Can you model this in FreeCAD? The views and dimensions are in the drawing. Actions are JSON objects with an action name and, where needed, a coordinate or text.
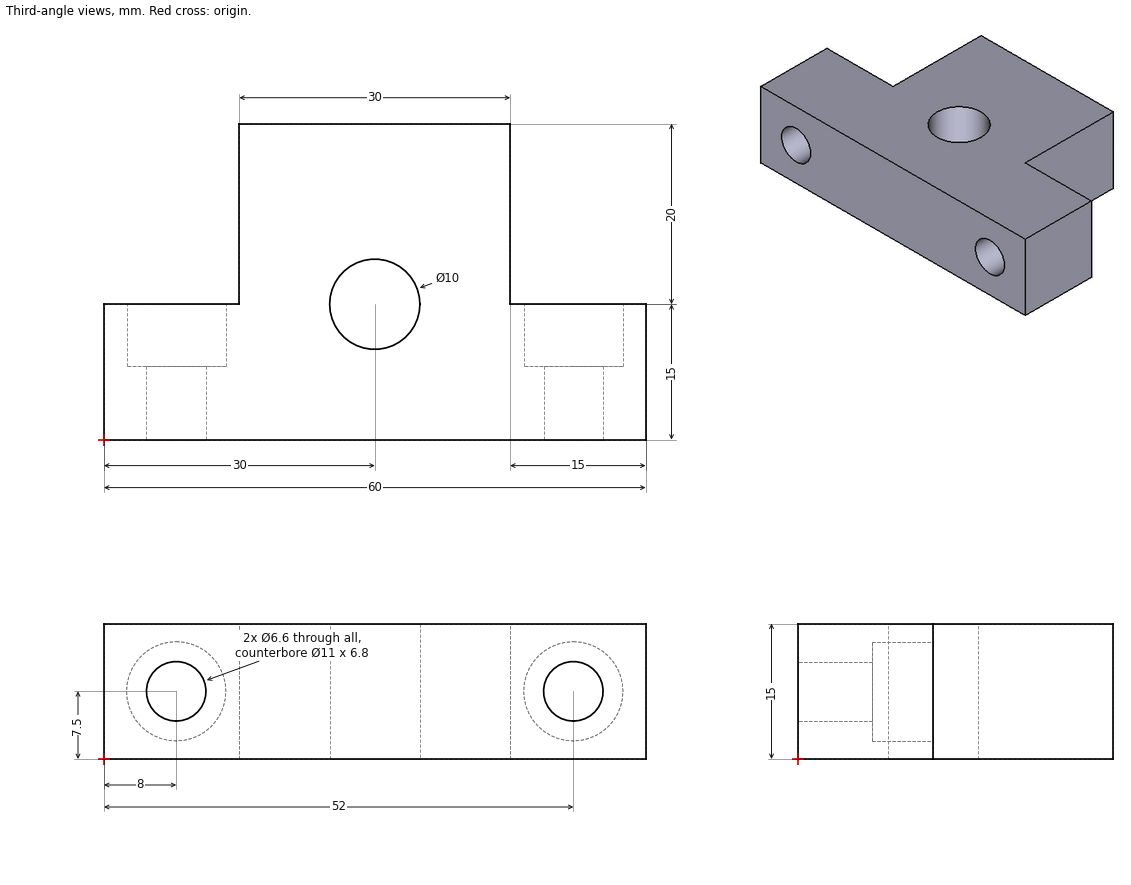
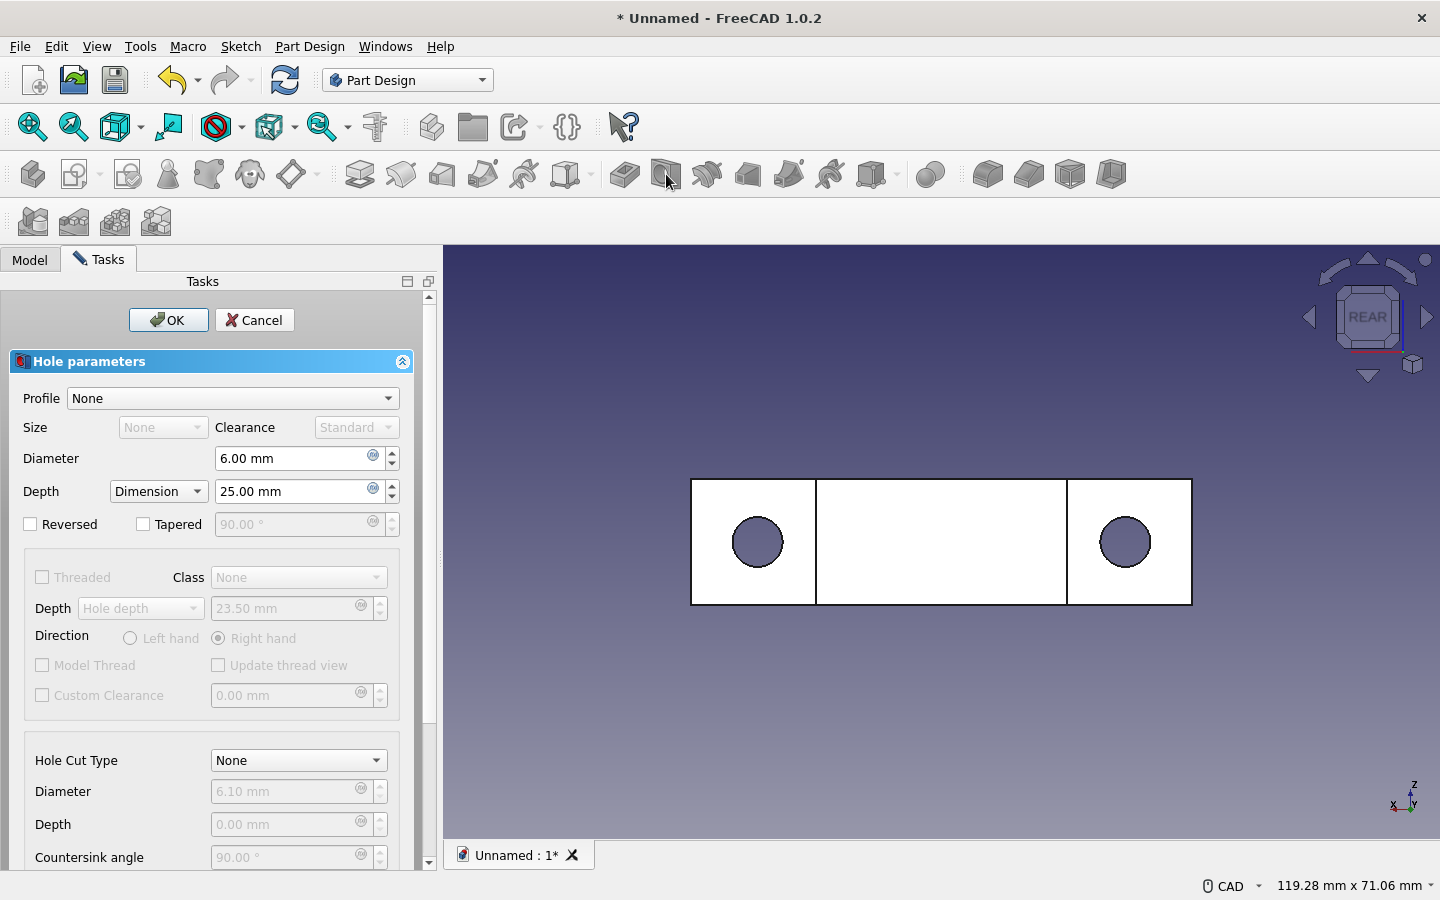
{"action": "triple_click", "coordinate": [300, 458]}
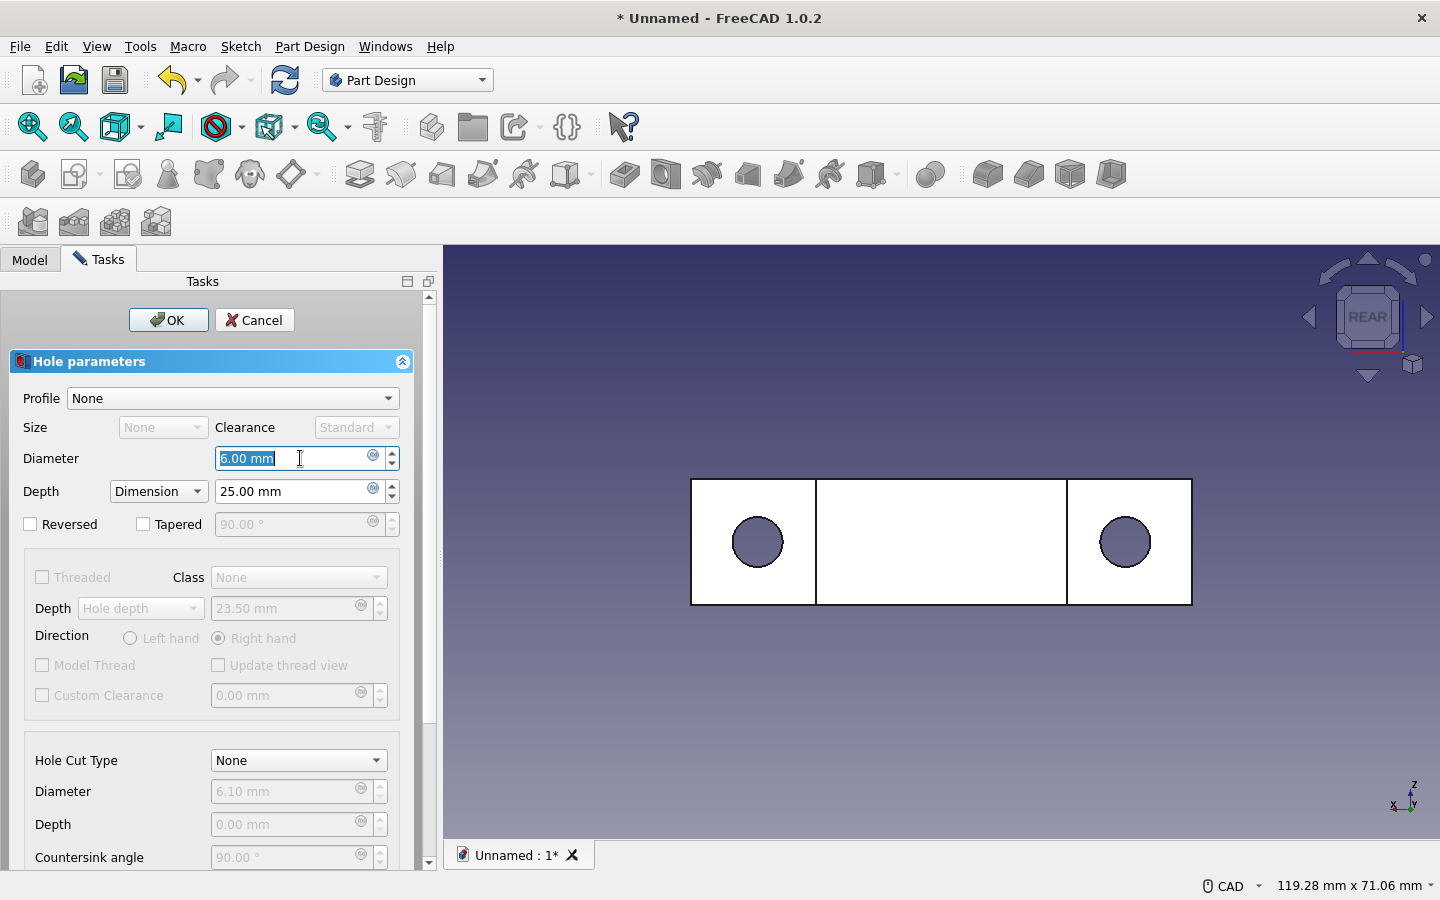
{"action": "type", "text": "6.6"}
{"action": "key", "text": "Tab"}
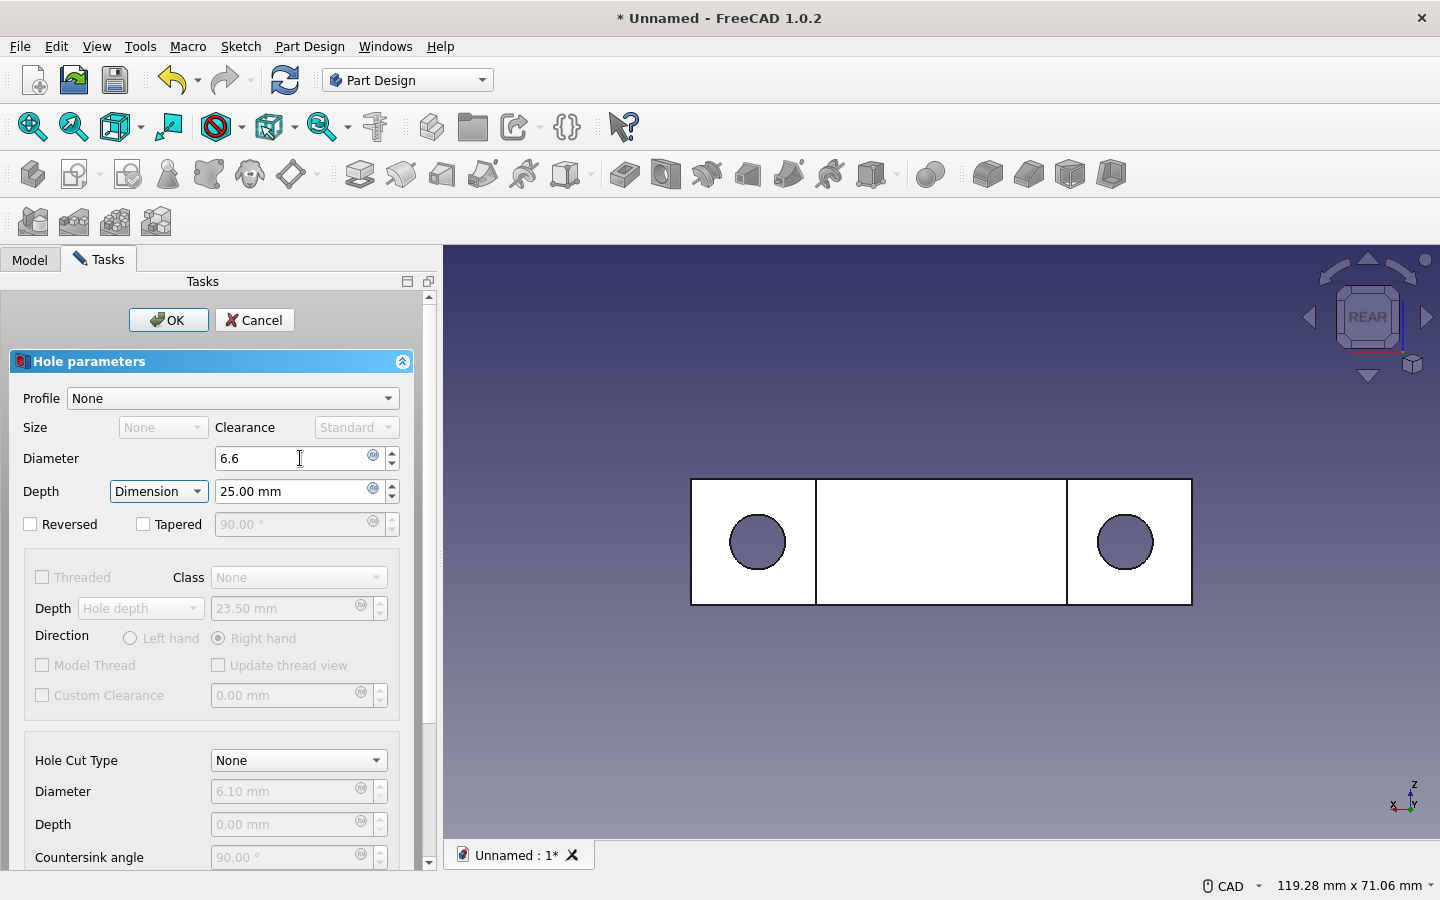
{"action": "left_click", "coordinate": [160, 492]}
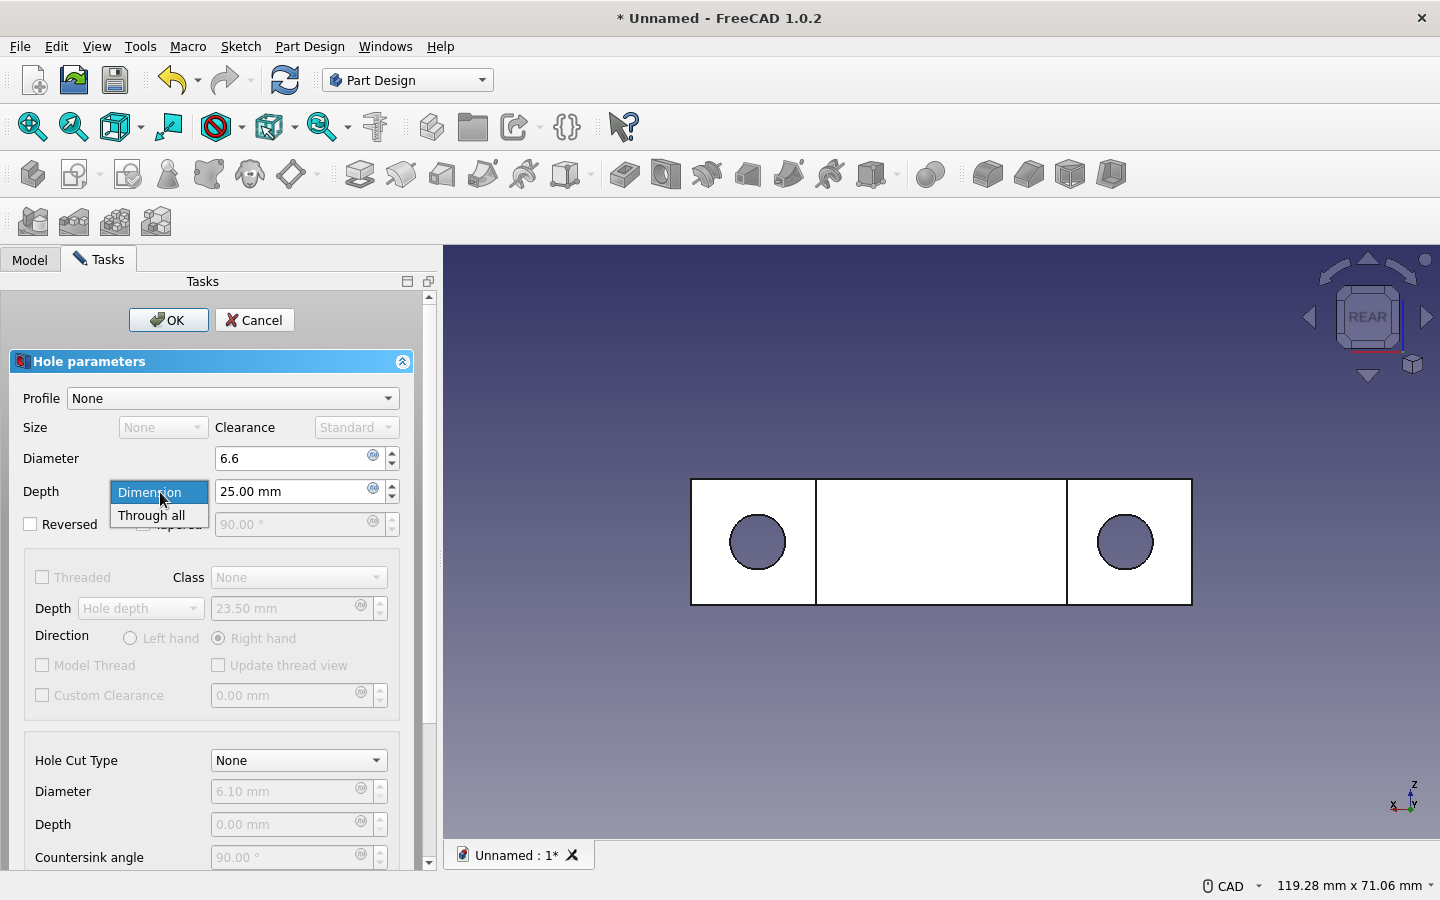
{"action": "left_click", "coordinate": [158, 516]}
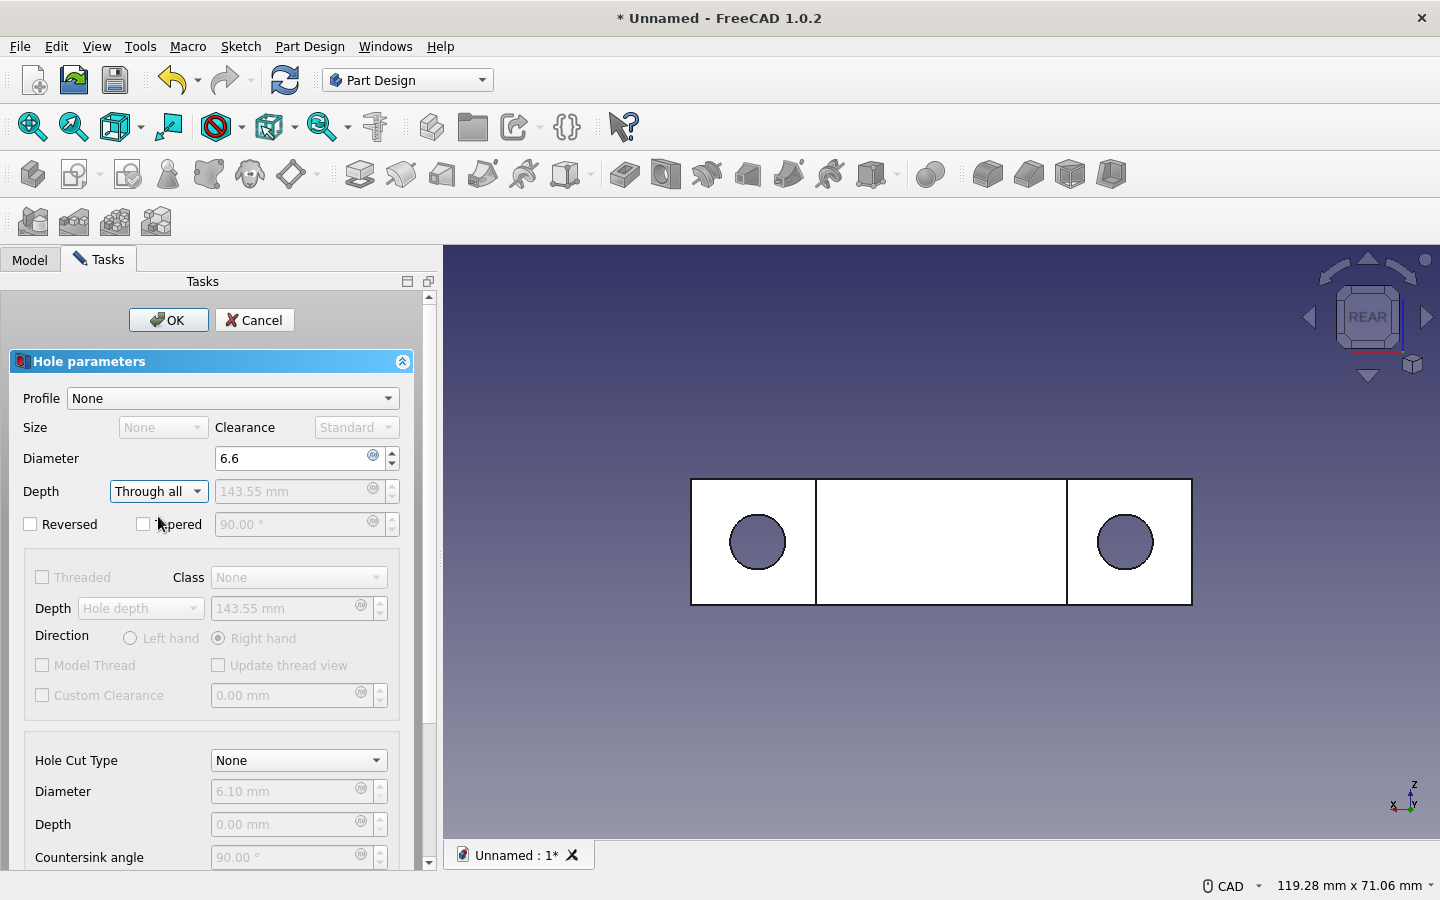
{"action": "left_click", "coordinate": [300, 760]}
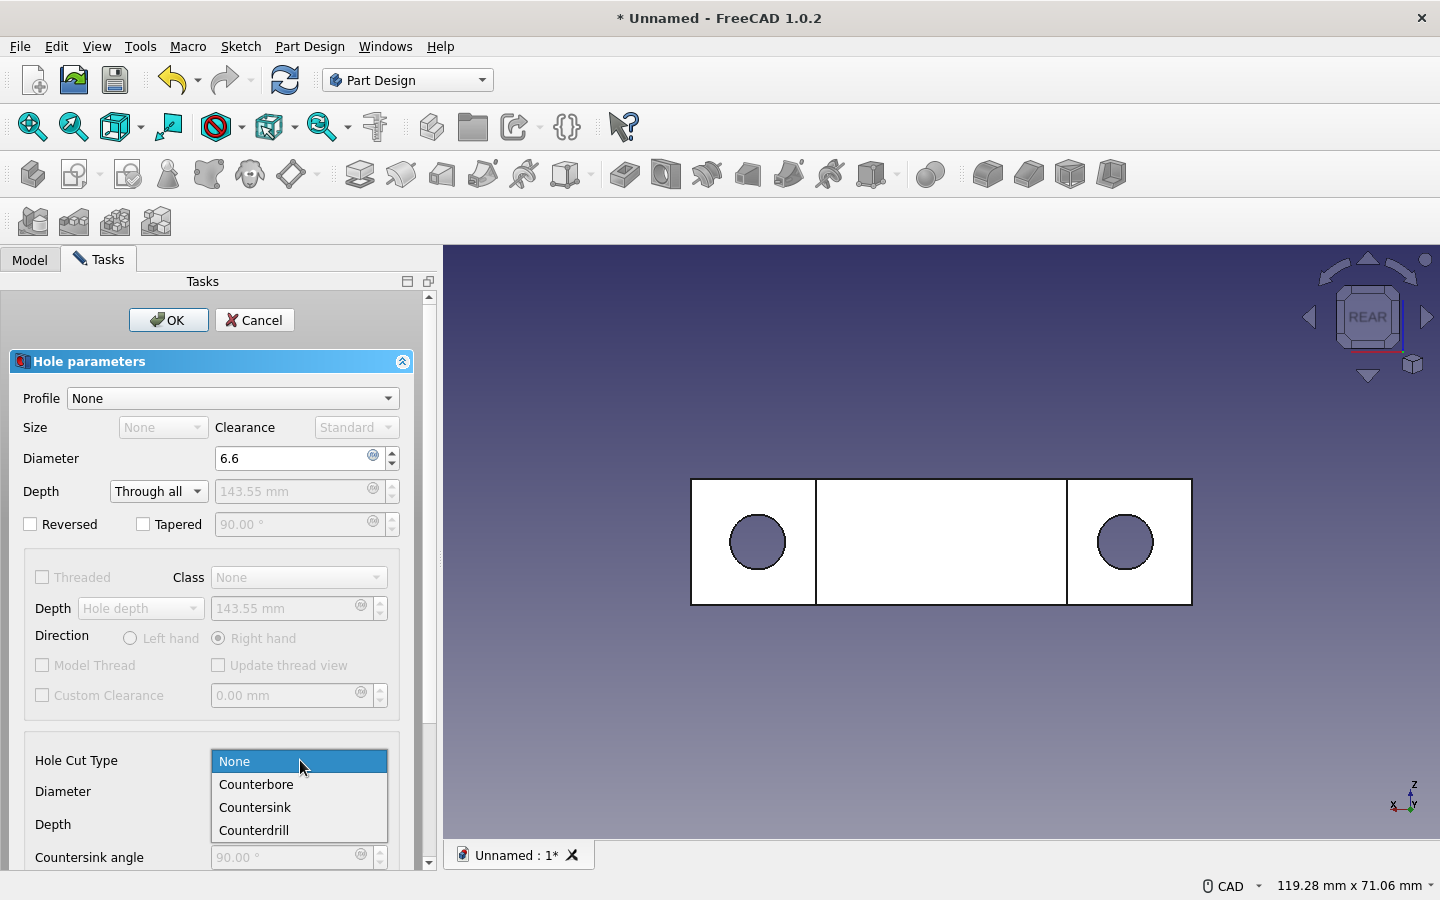
{"action": "left_click", "coordinate": [298, 784]}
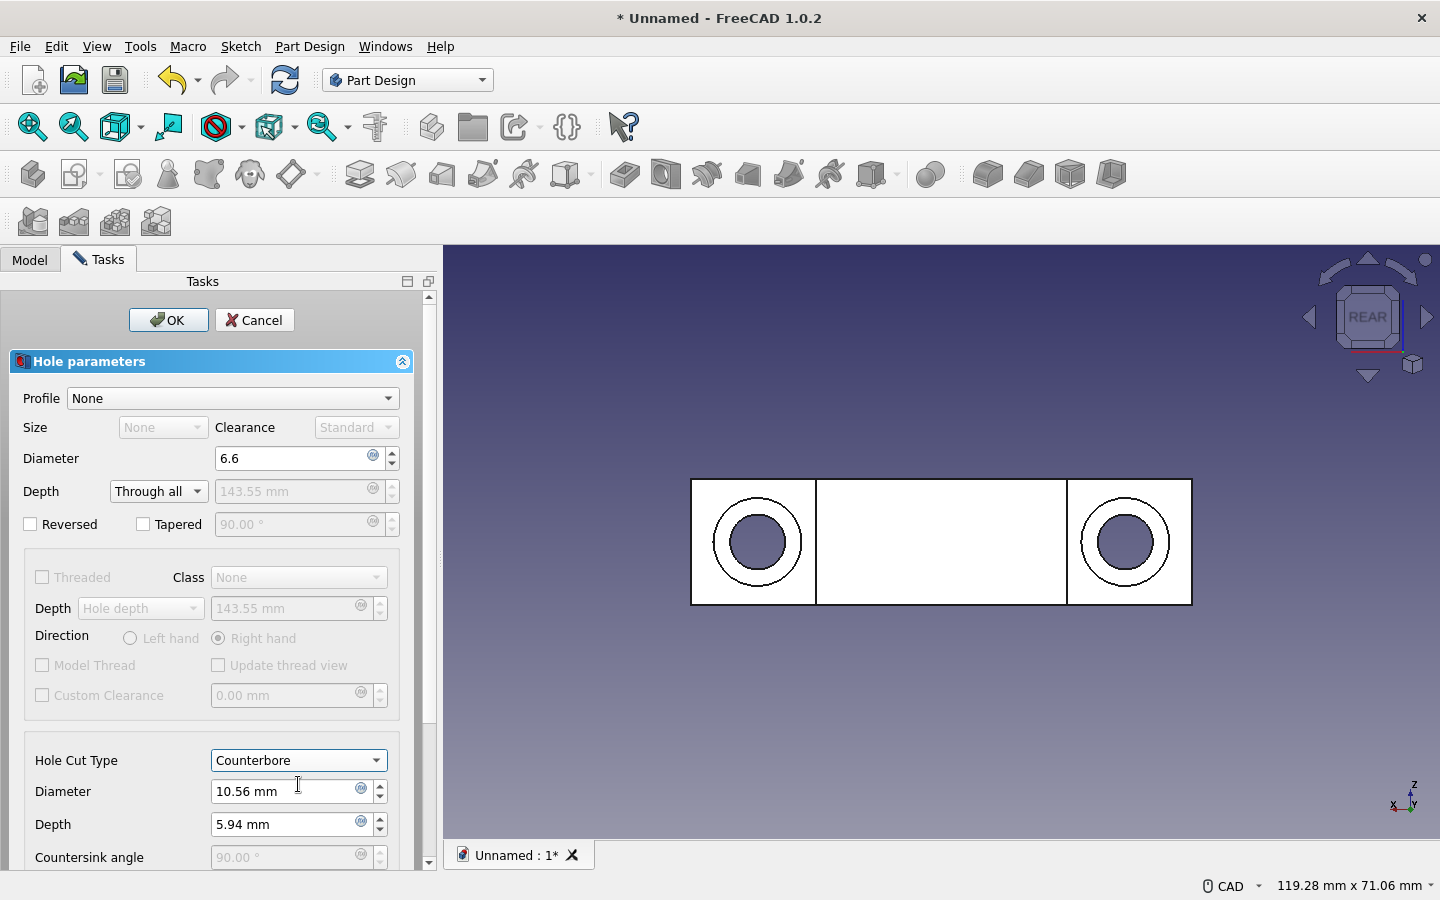
{"action": "triple_click", "coordinate": [292, 792]}